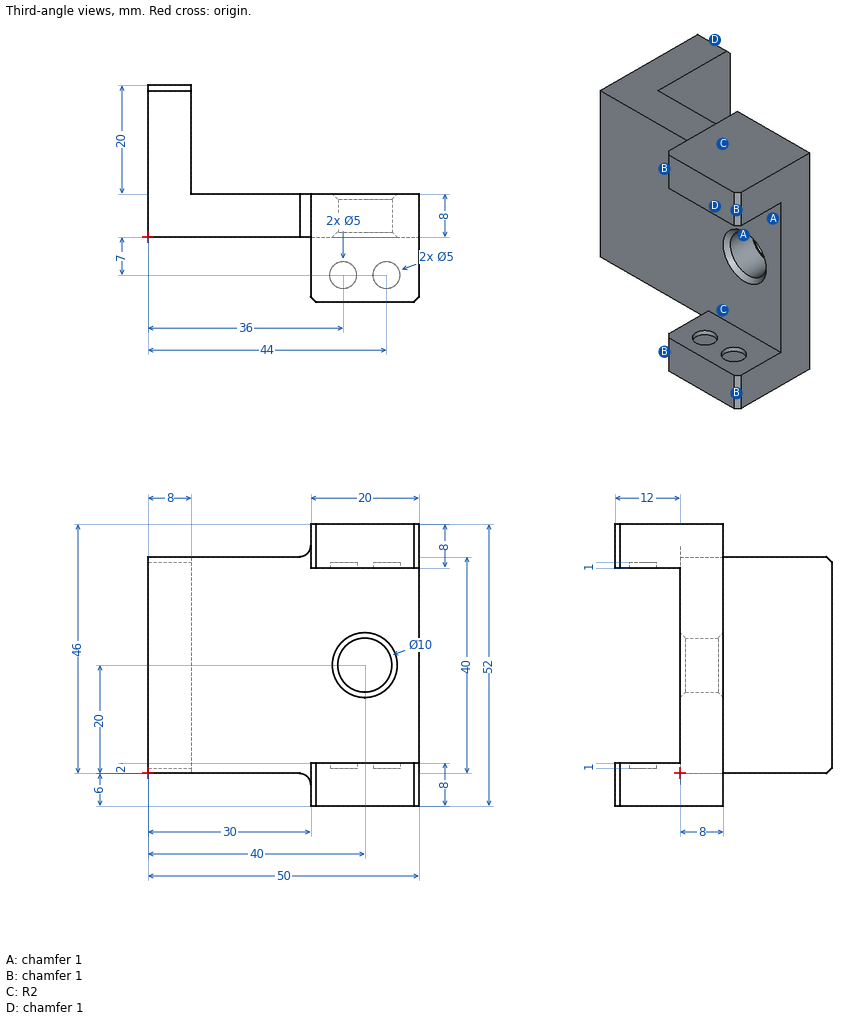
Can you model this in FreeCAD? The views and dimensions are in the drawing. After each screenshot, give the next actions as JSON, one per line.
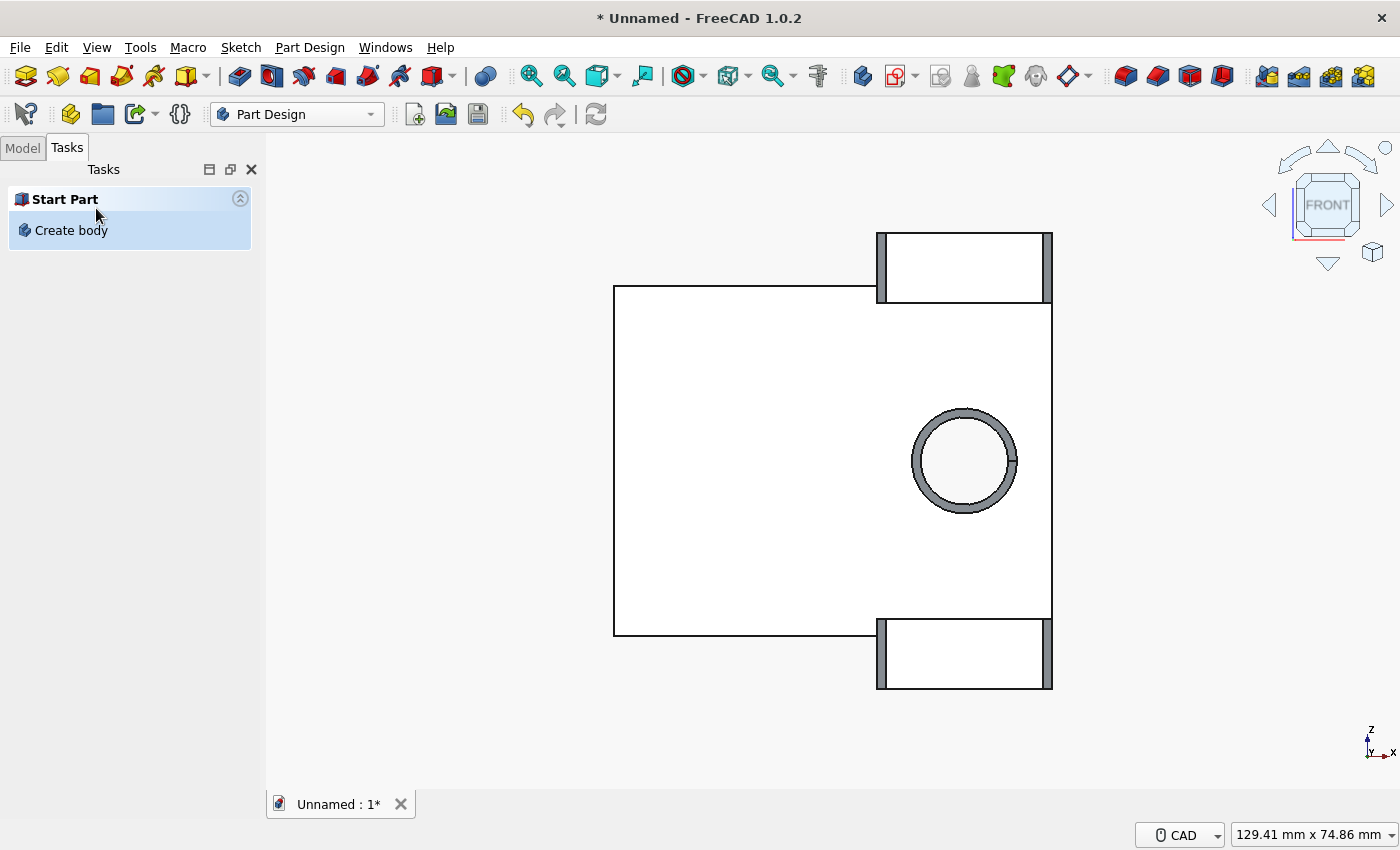
{"action": "key", "text": "0"}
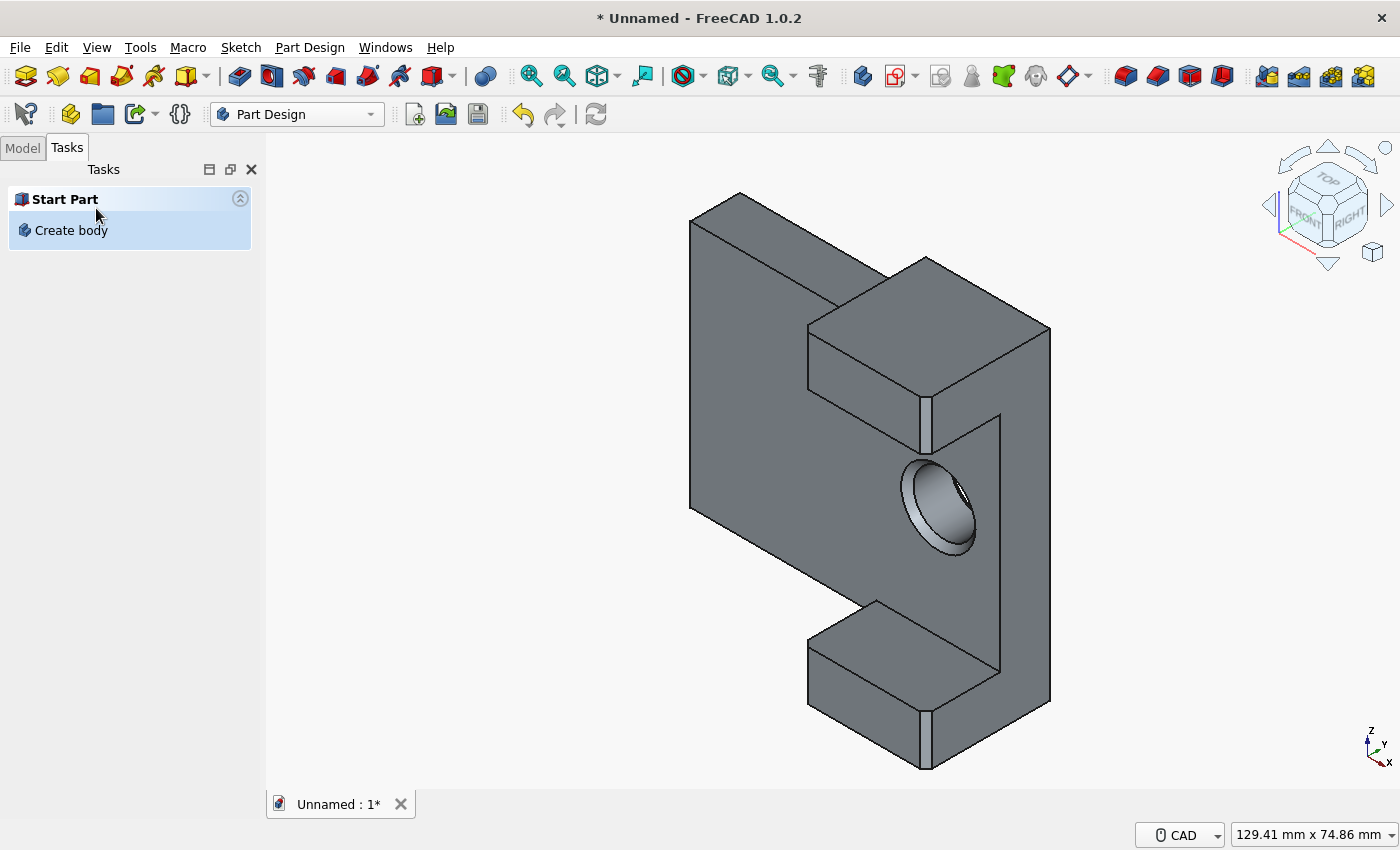
{"action": "key", "text": "2"}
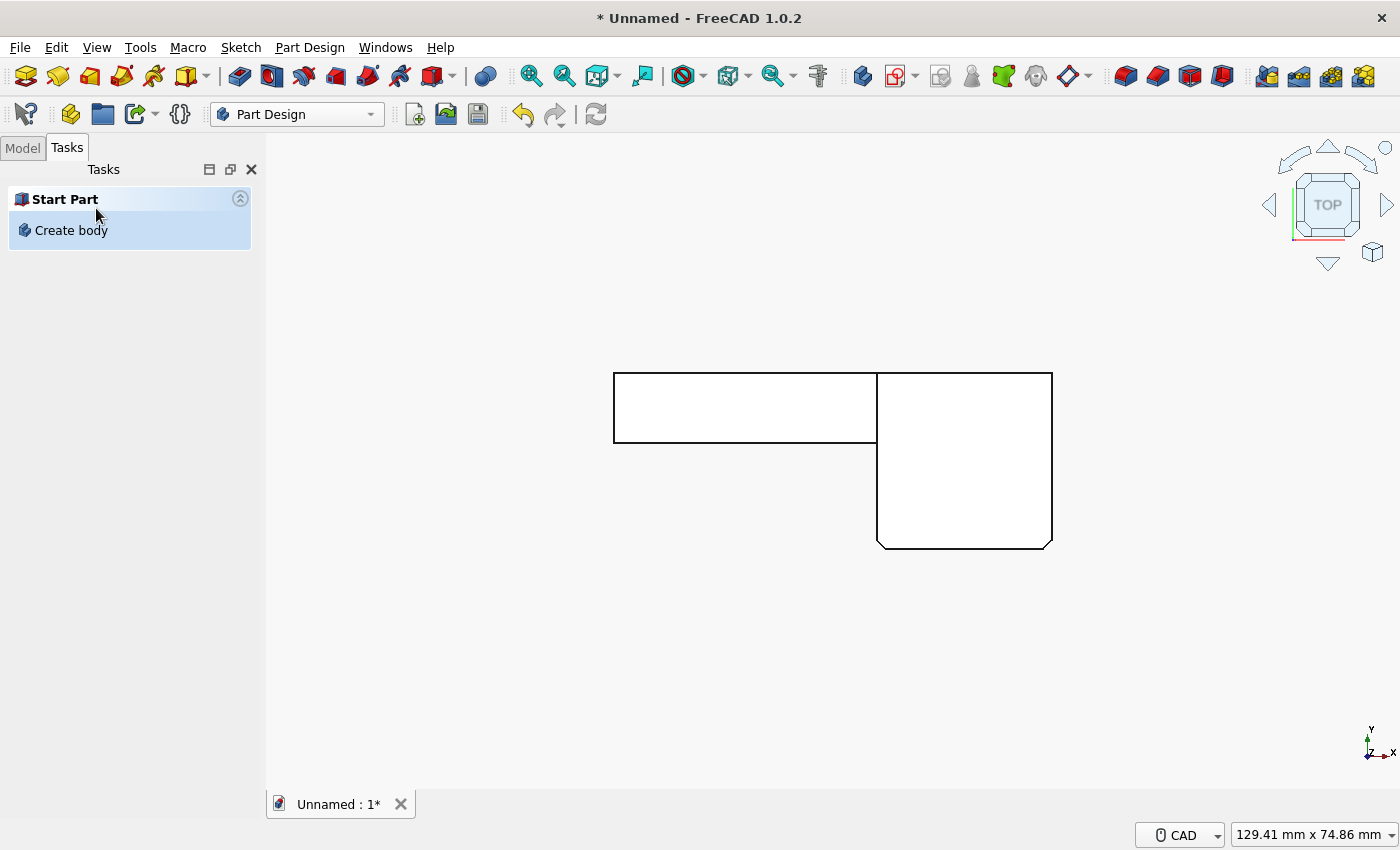
{"action": "left_click", "coordinate": [532, 76]}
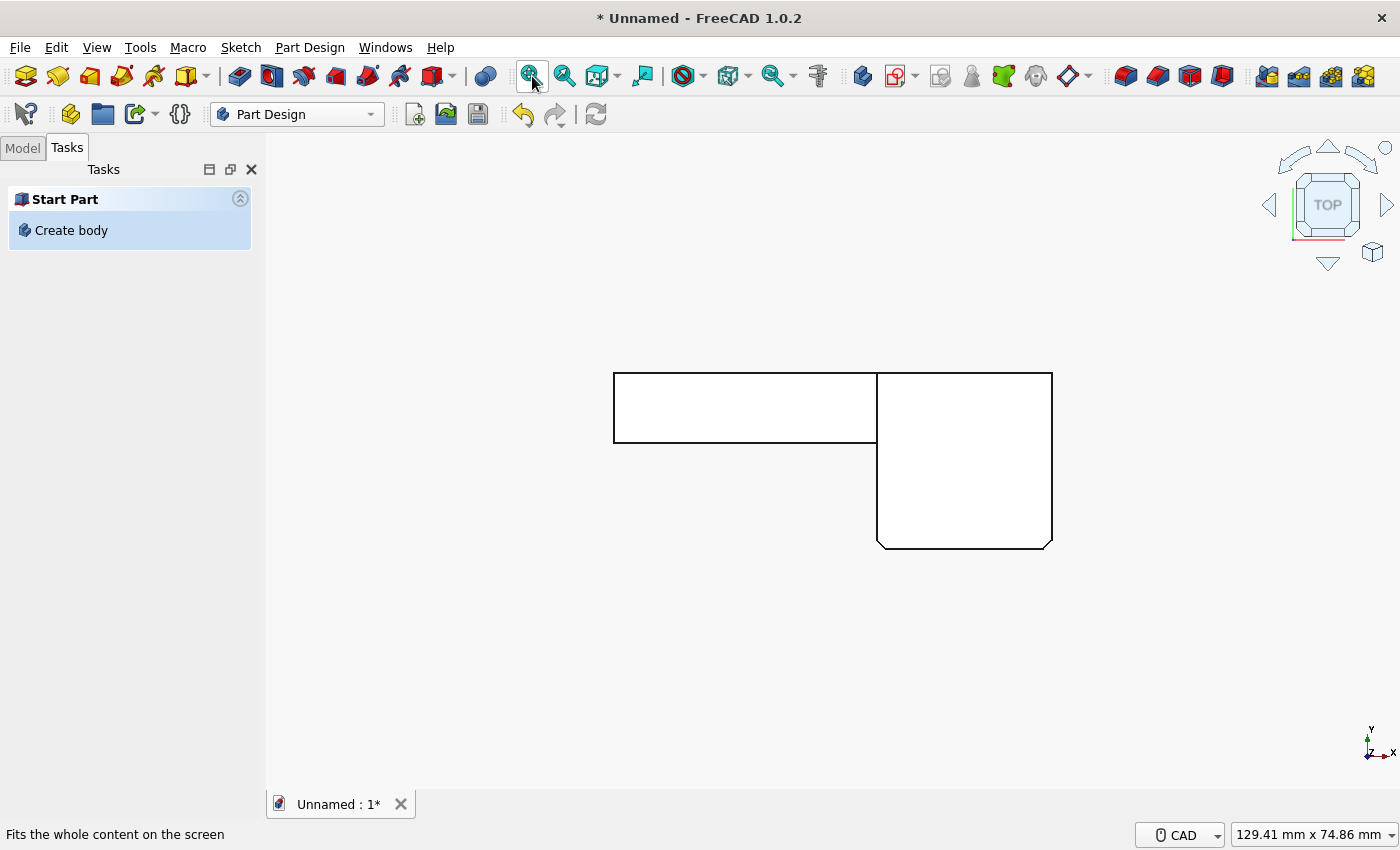
{"action": "key", "text": "1"}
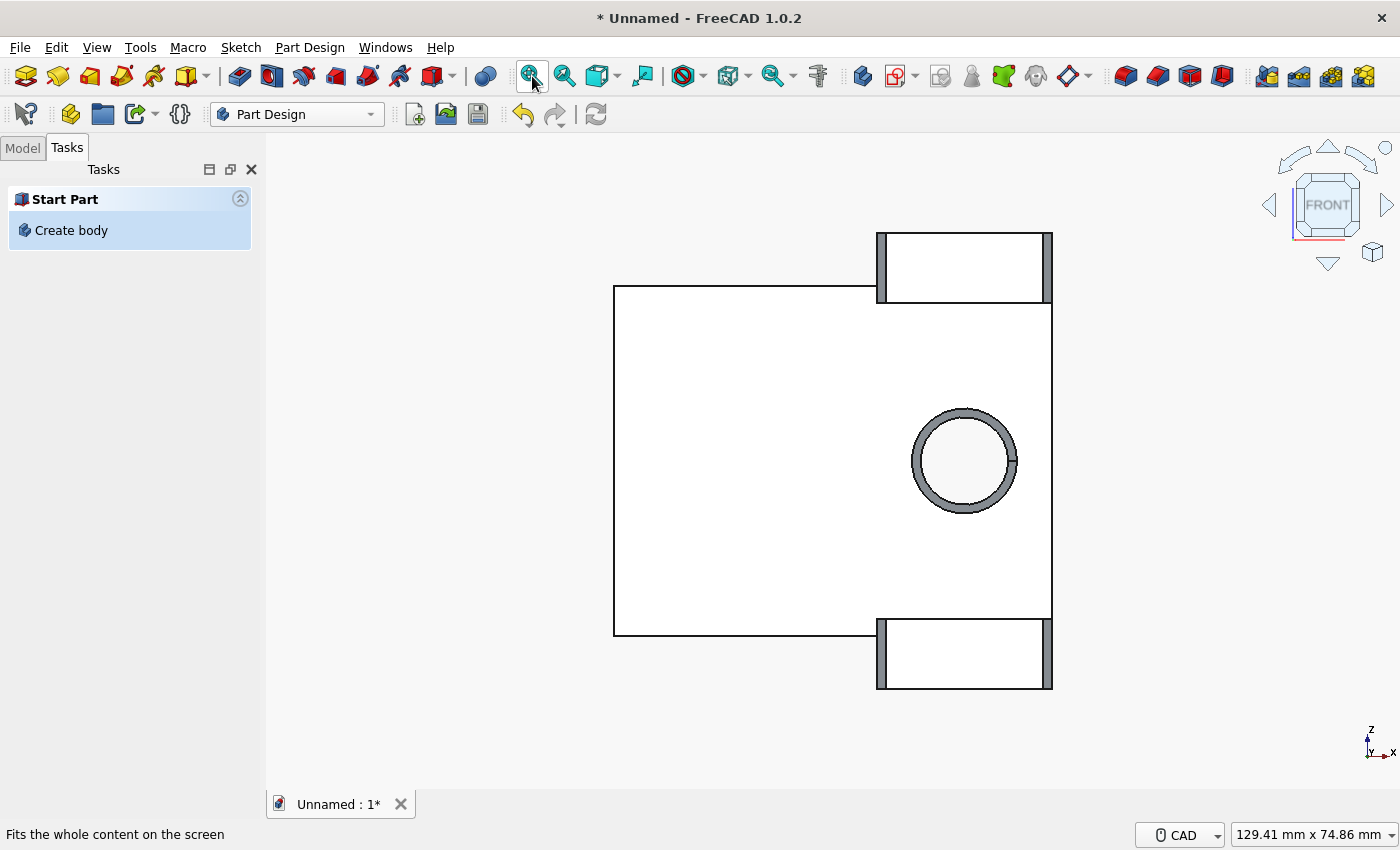
{"action": "key", "text": "3"}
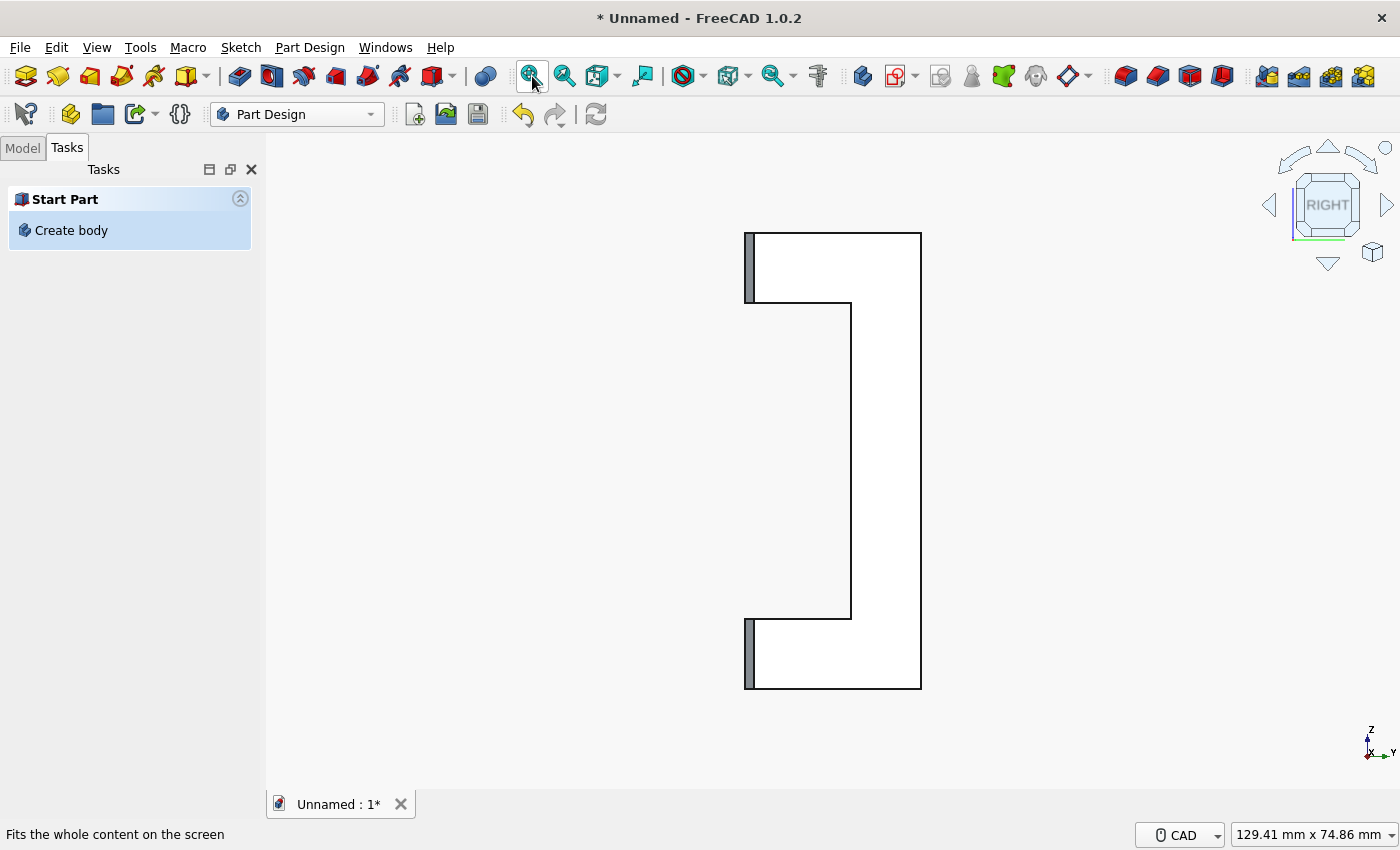
{"action": "key", "text": "5"}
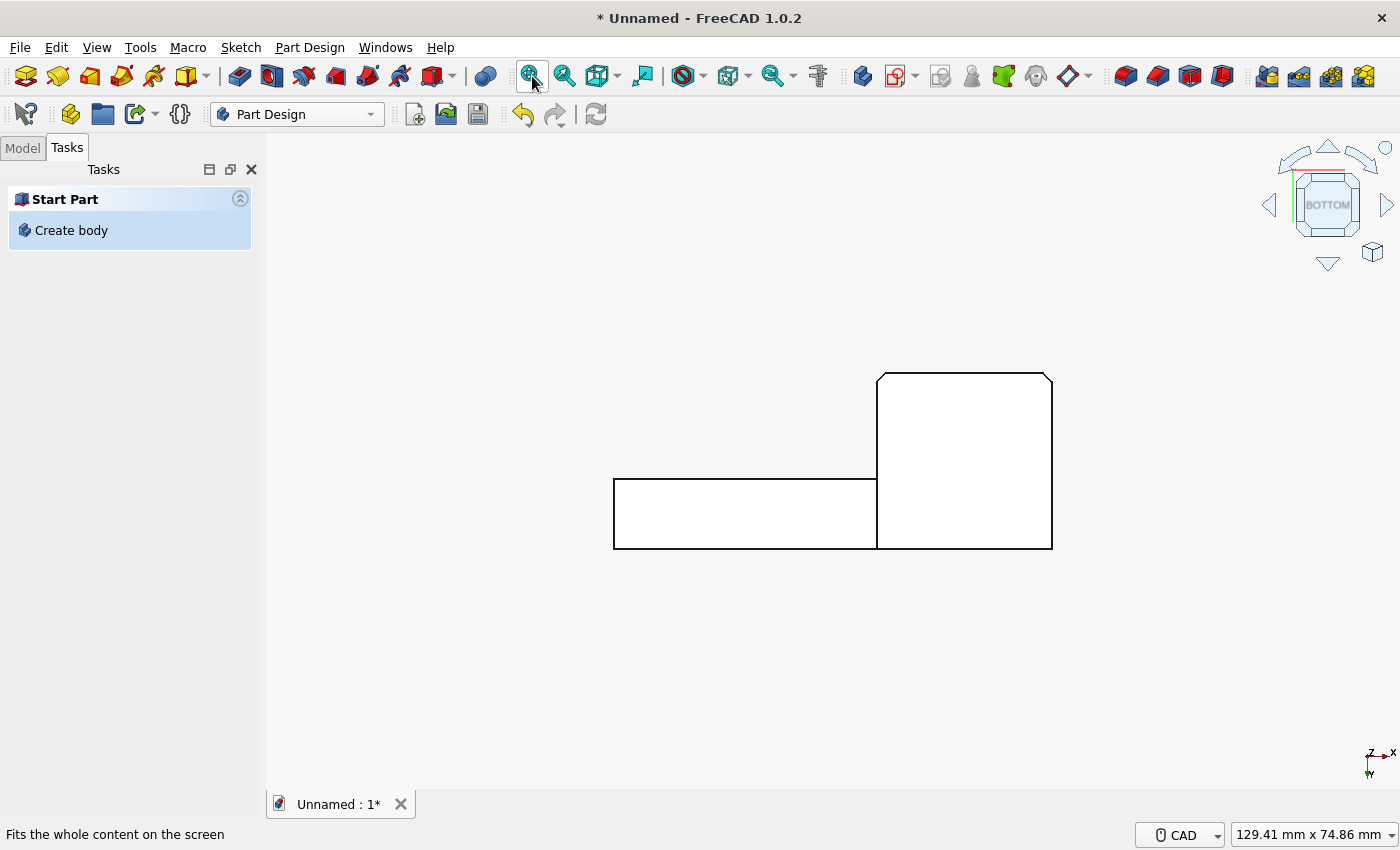
{"action": "left_click", "coordinate": [532, 76]}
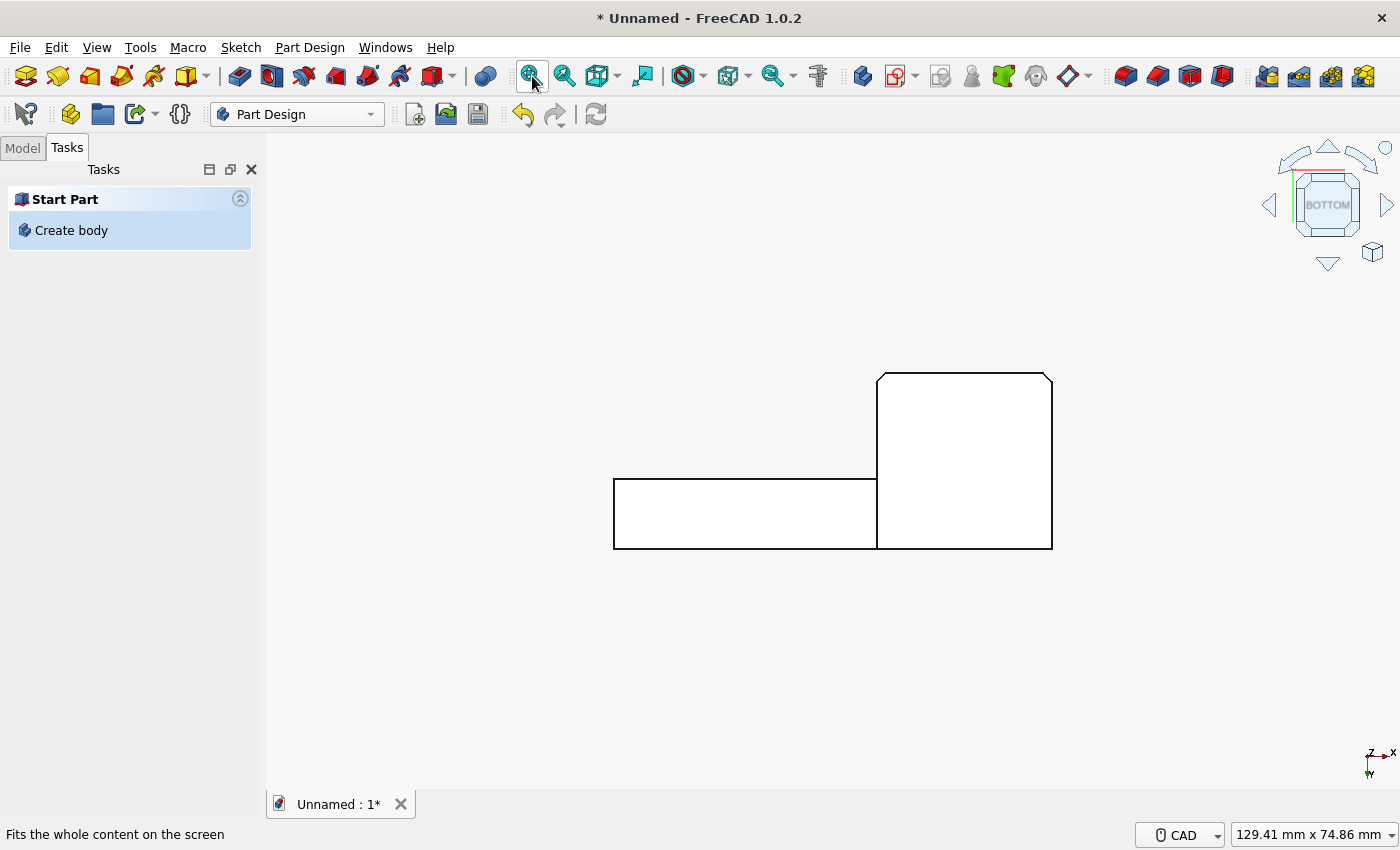
{"action": "key", "text": "4"}